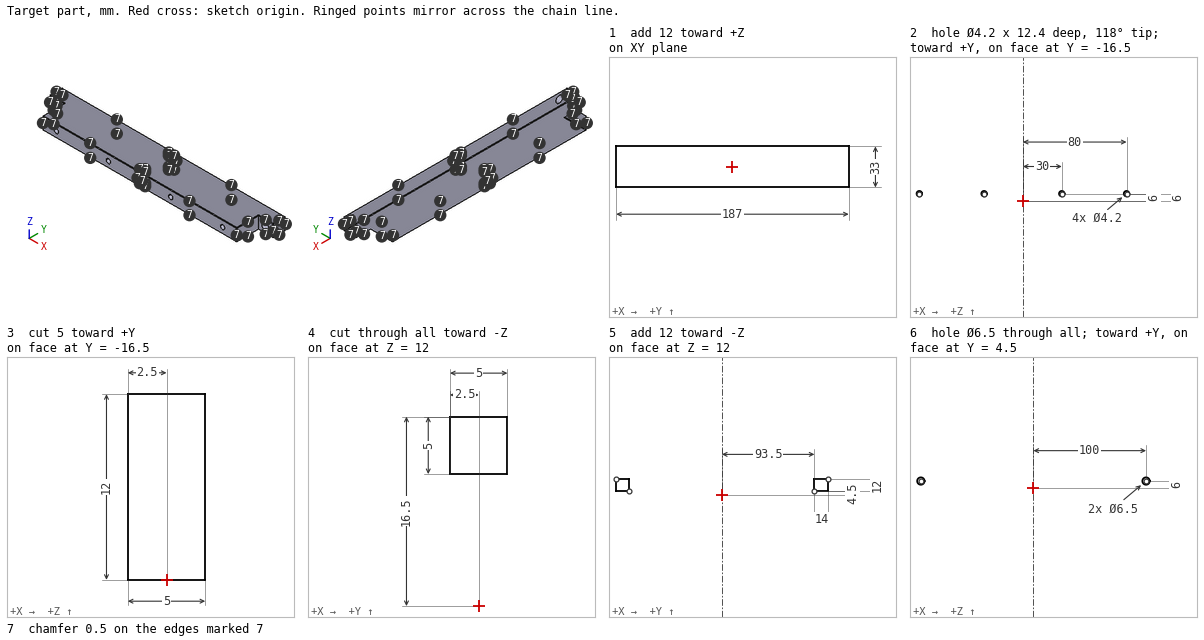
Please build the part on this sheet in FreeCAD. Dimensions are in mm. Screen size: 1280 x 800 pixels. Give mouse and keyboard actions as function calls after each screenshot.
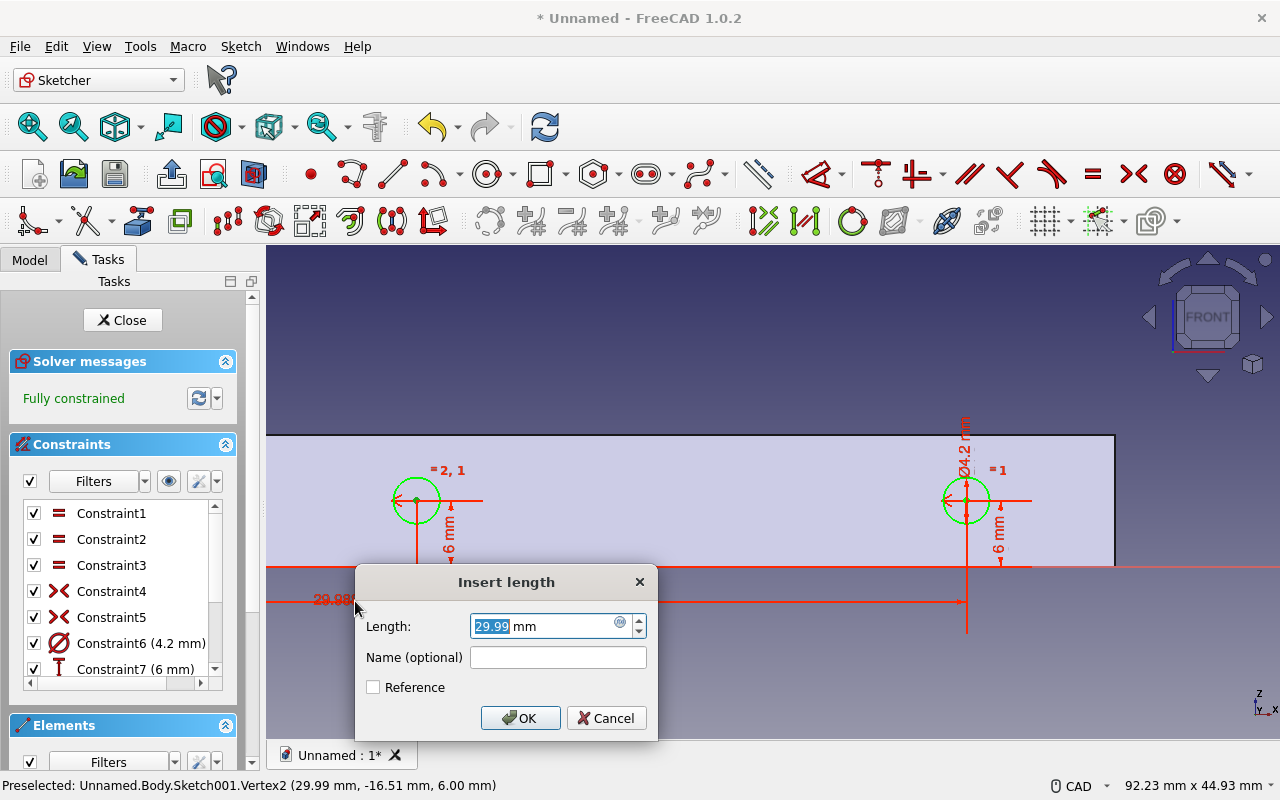
text(30)
key(Return)
key(Escape)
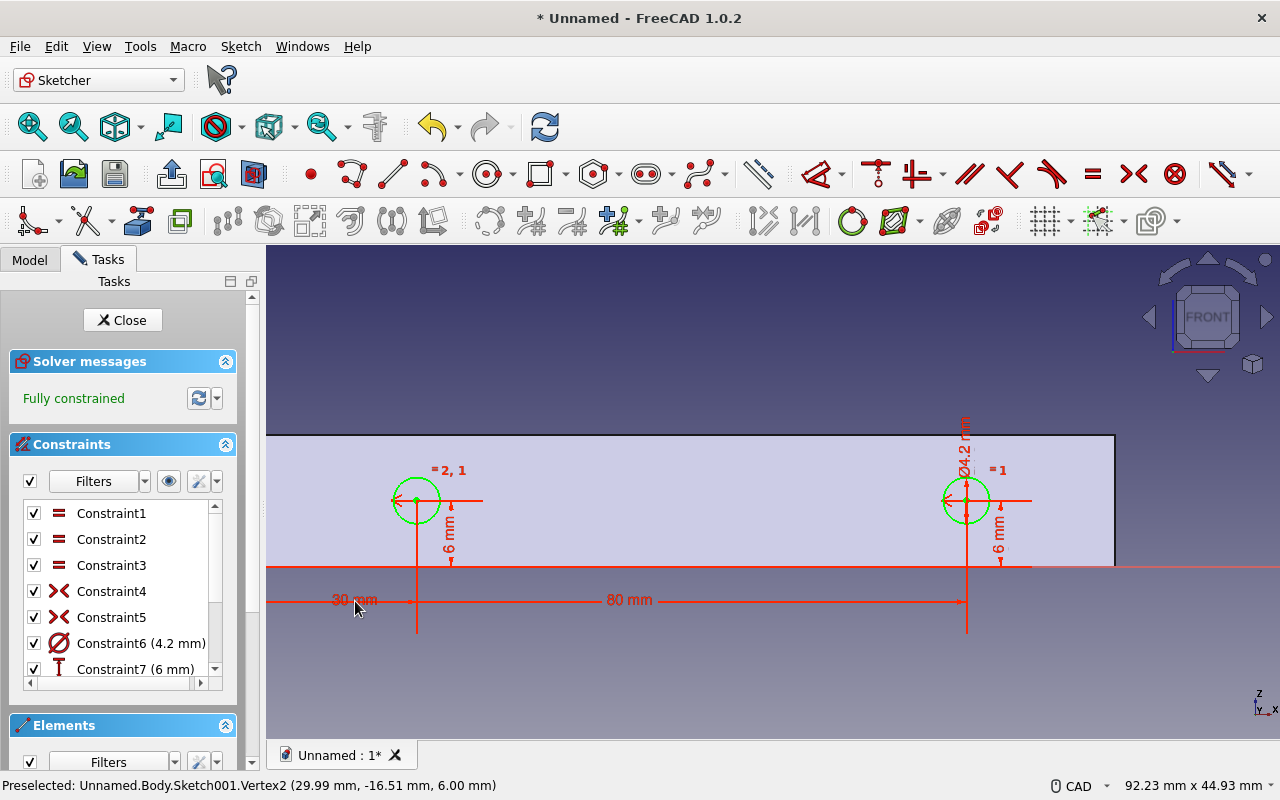
click(123, 320)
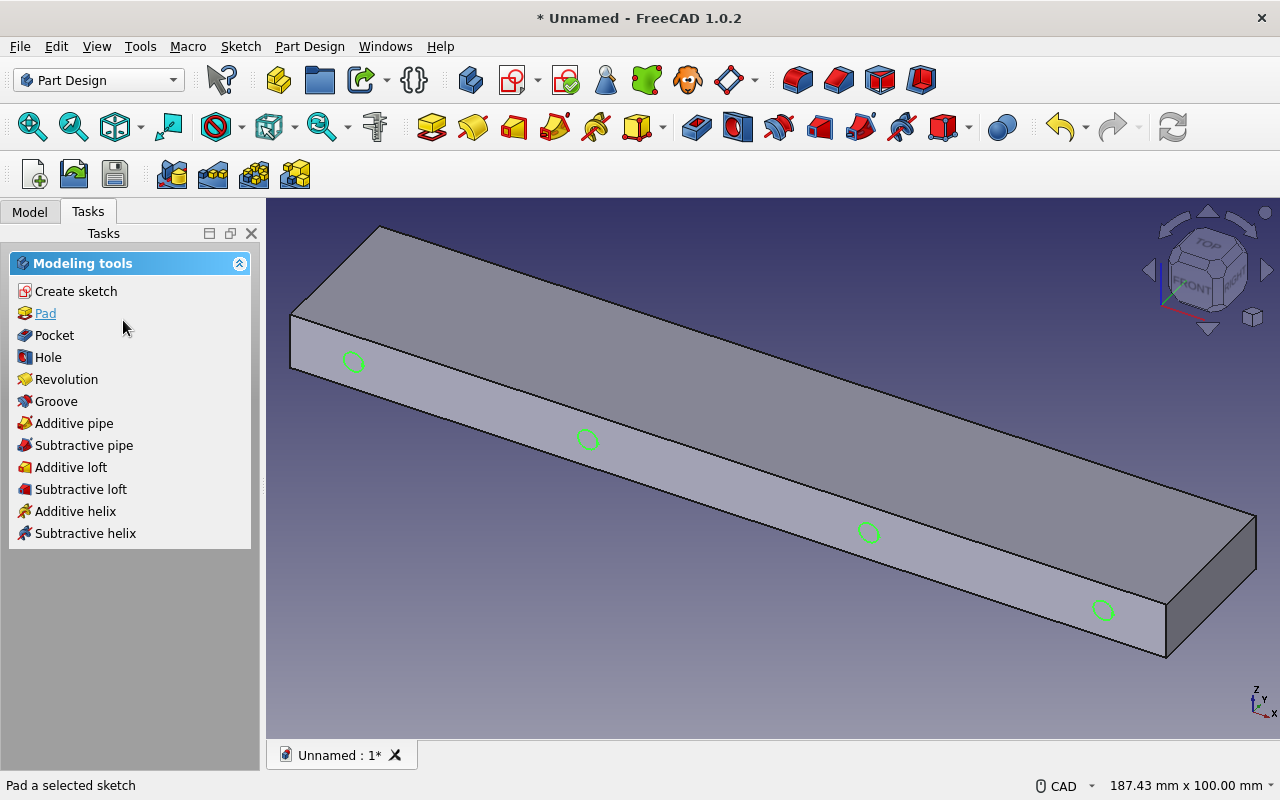
click(738, 128)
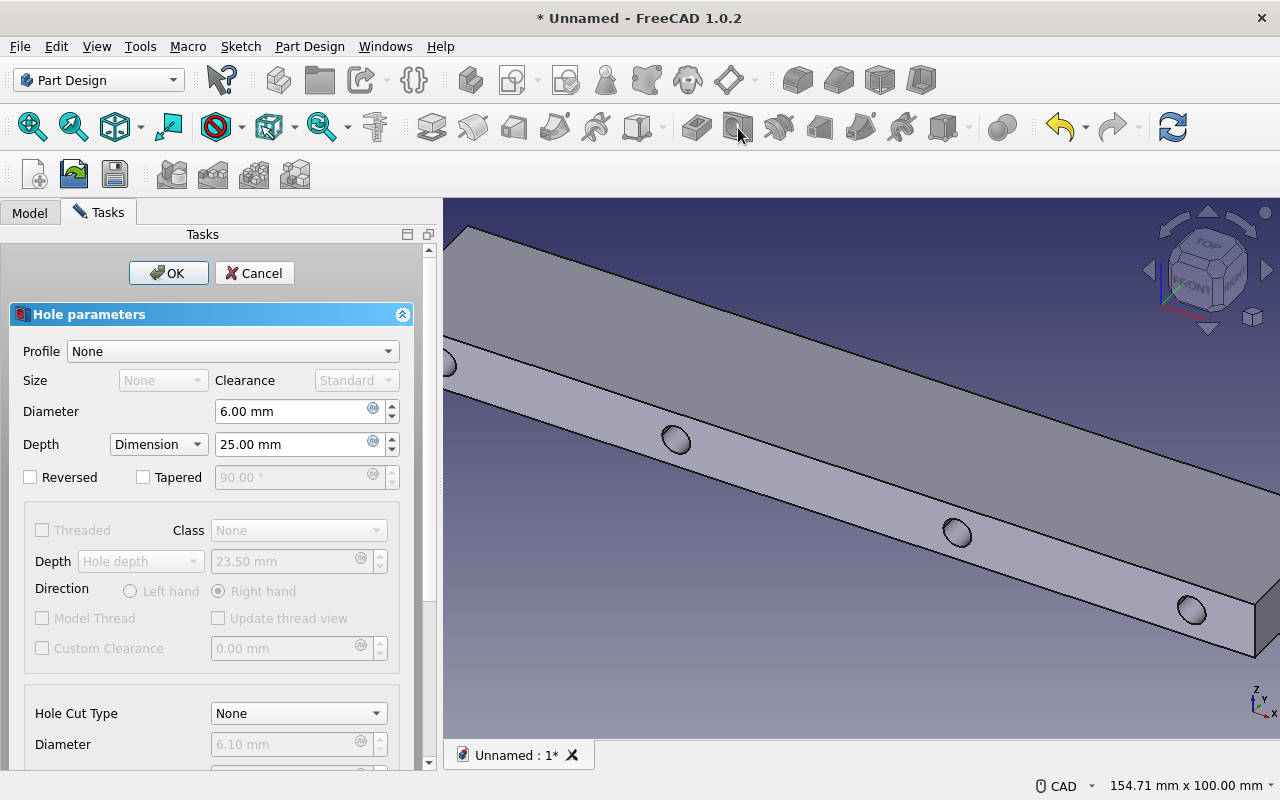
triple_click(300, 412)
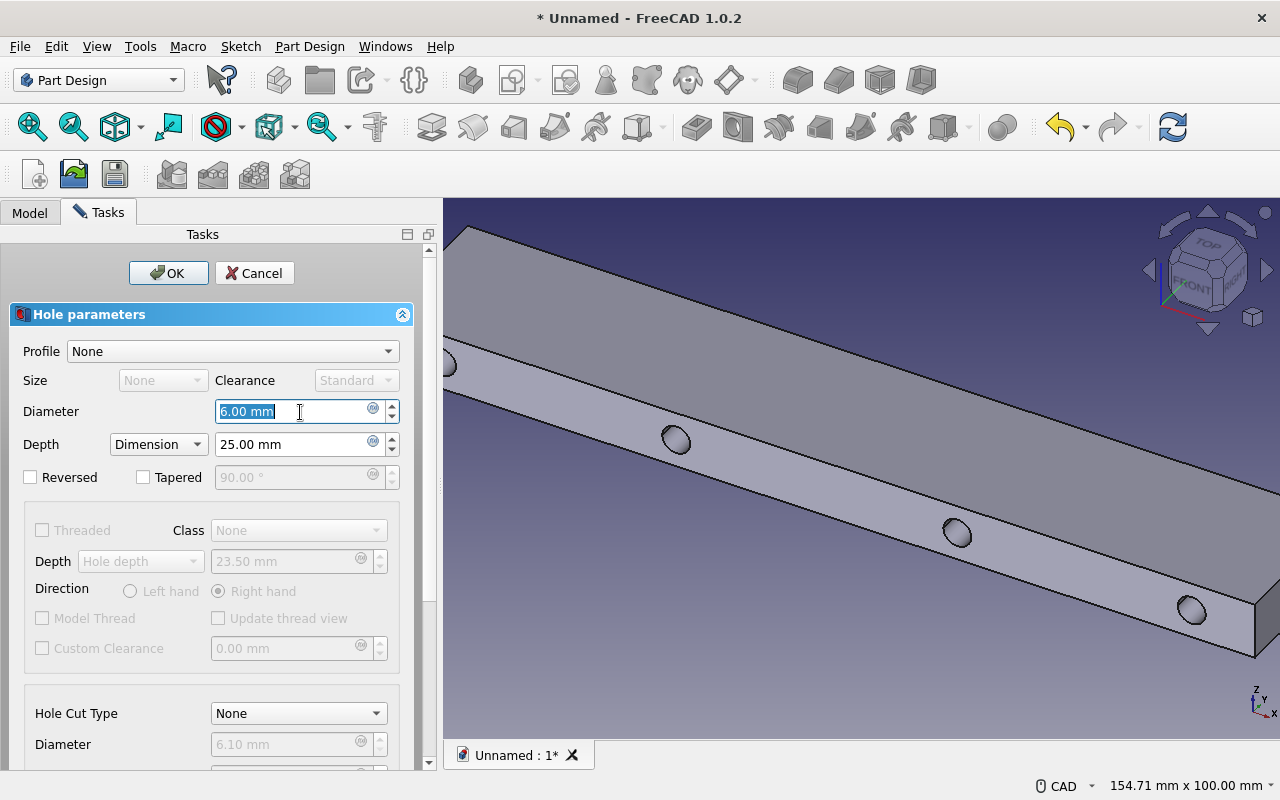
text(4.2)
key(Tab)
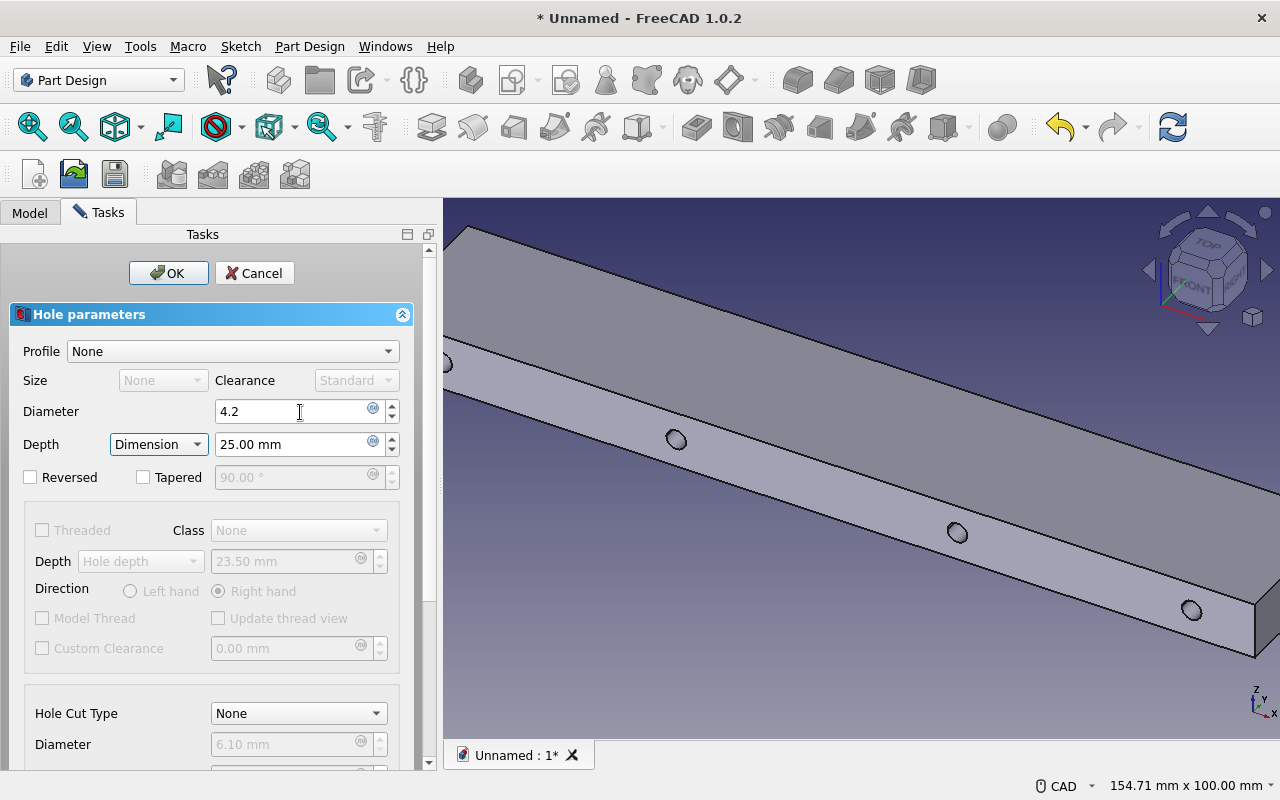
triple_click(300, 444)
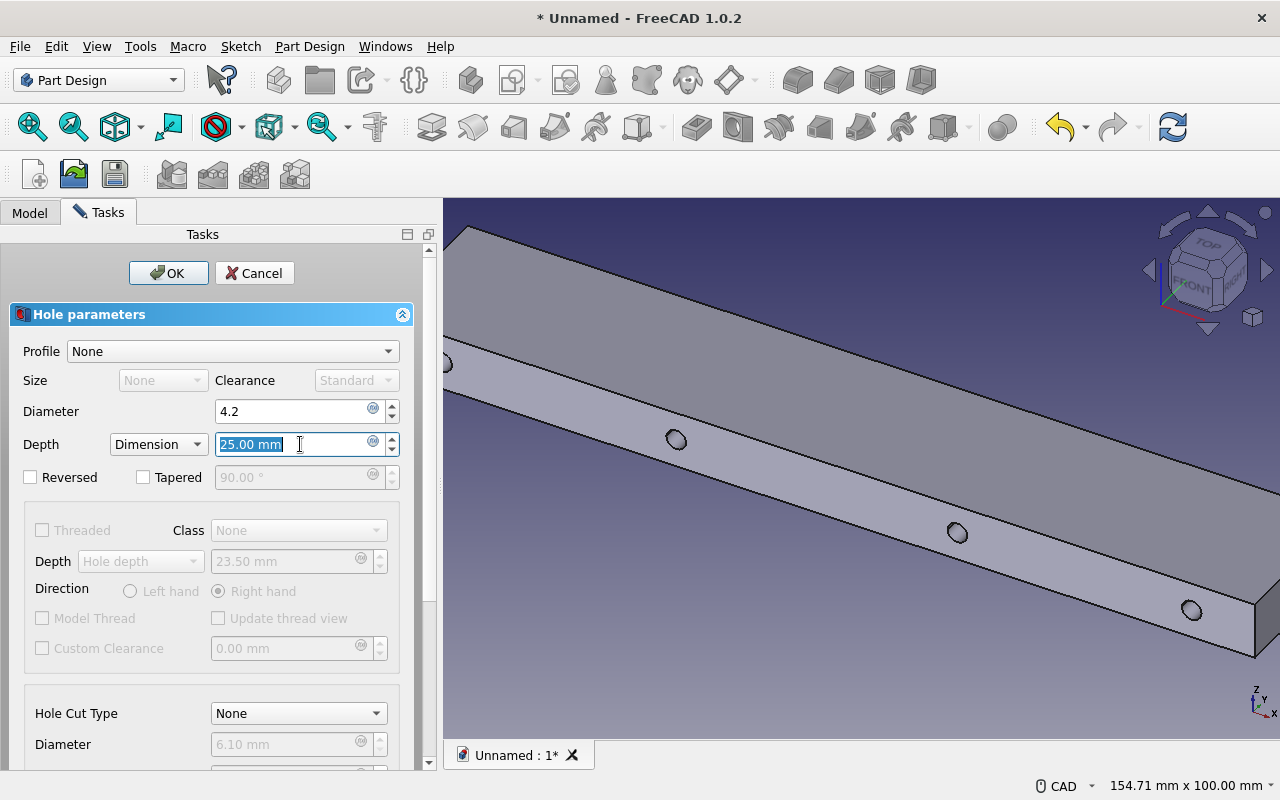
text(12.4)
key(Tab)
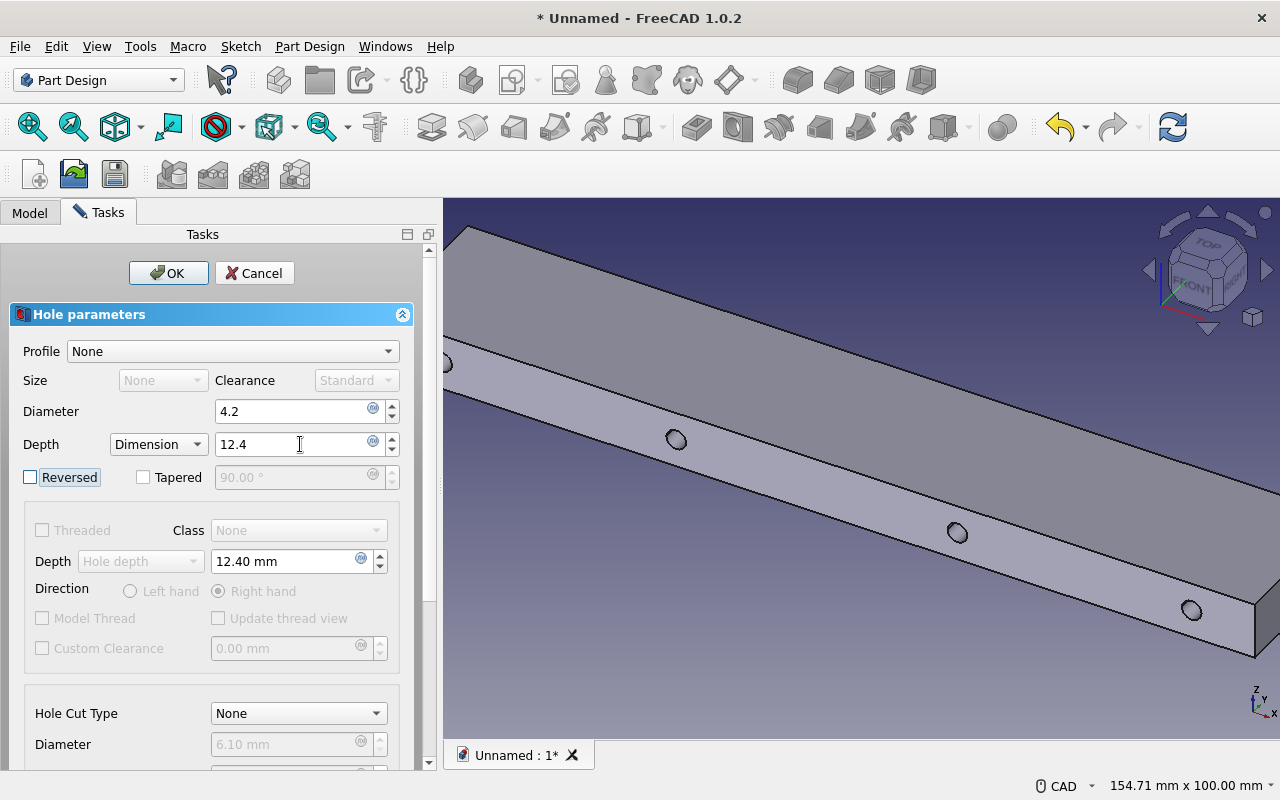
click(169, 273)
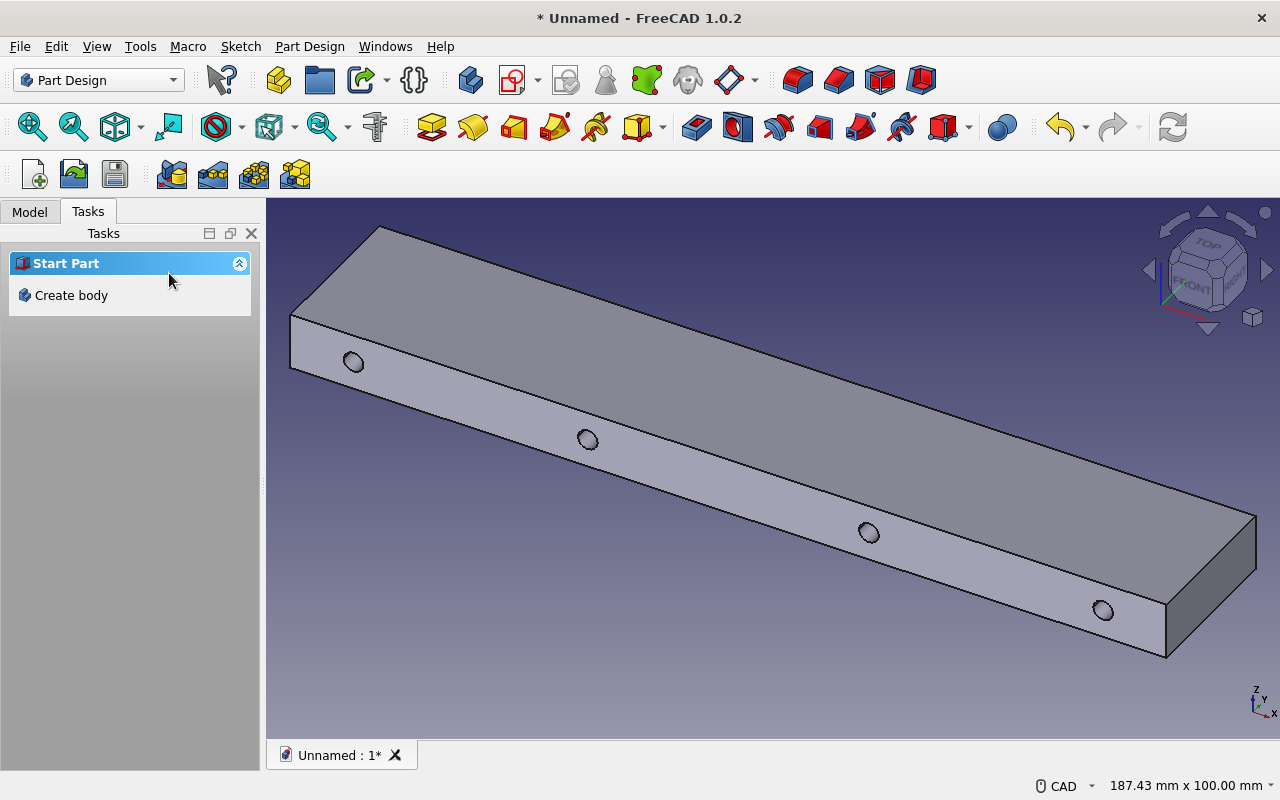
click(979, 568)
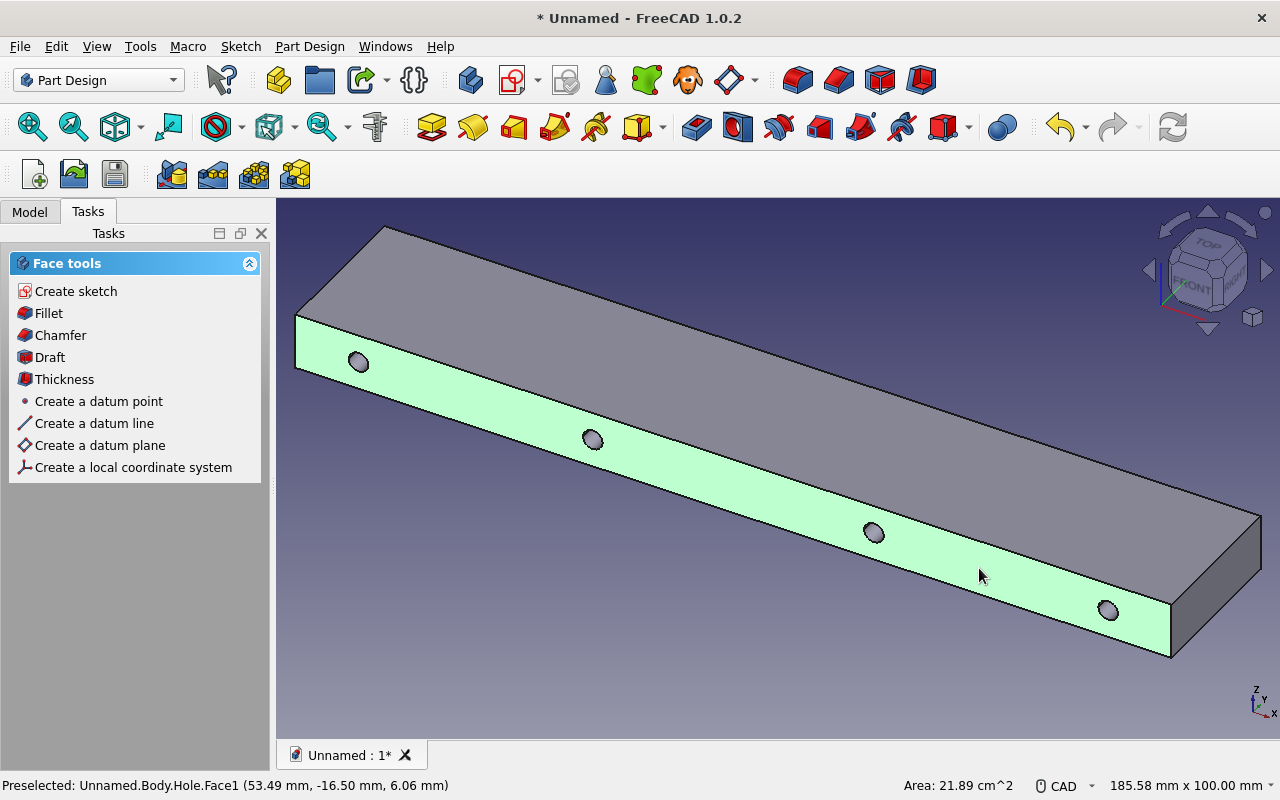
click(512, 80)